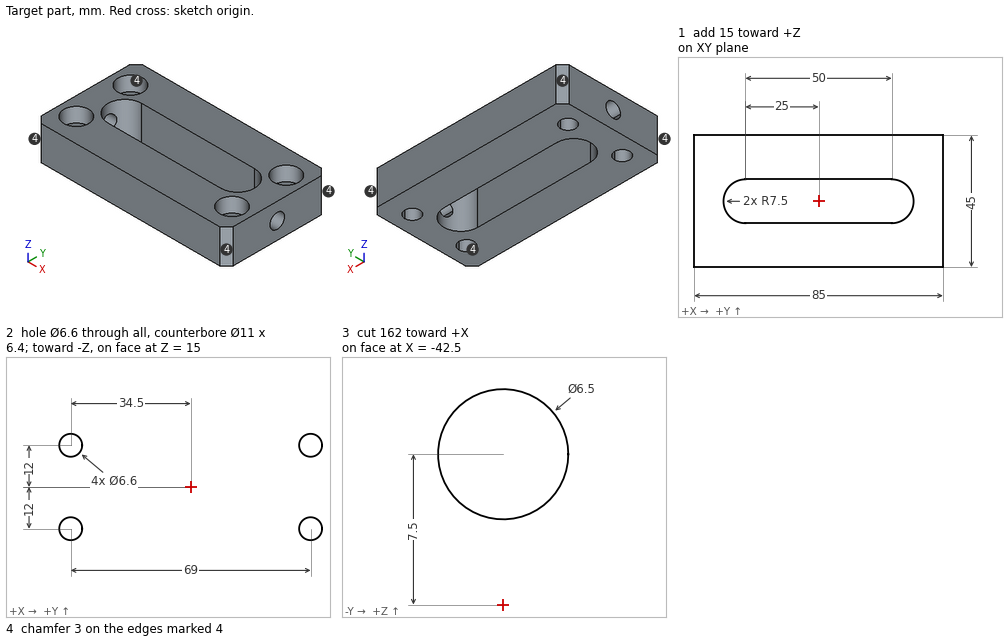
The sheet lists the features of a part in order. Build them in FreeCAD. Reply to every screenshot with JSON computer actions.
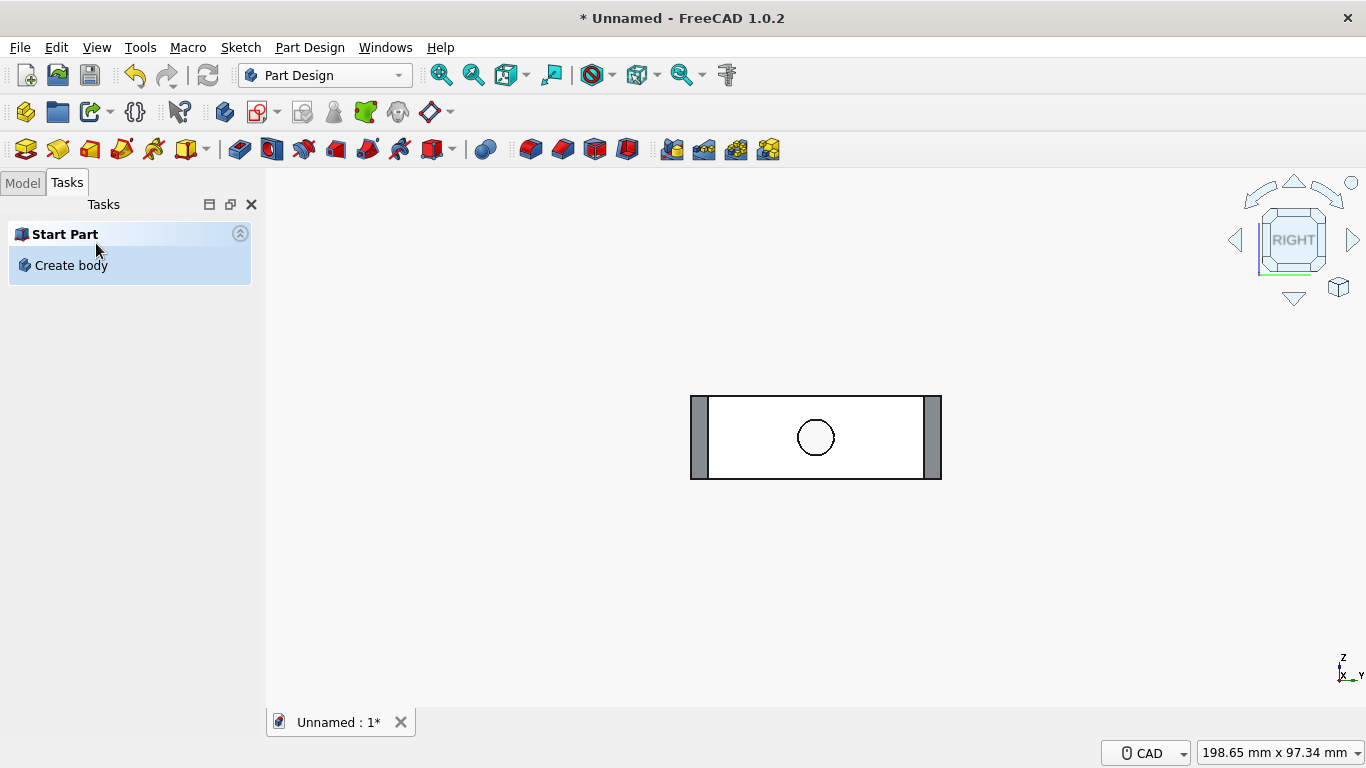
{"action": "key", "text": "0"}